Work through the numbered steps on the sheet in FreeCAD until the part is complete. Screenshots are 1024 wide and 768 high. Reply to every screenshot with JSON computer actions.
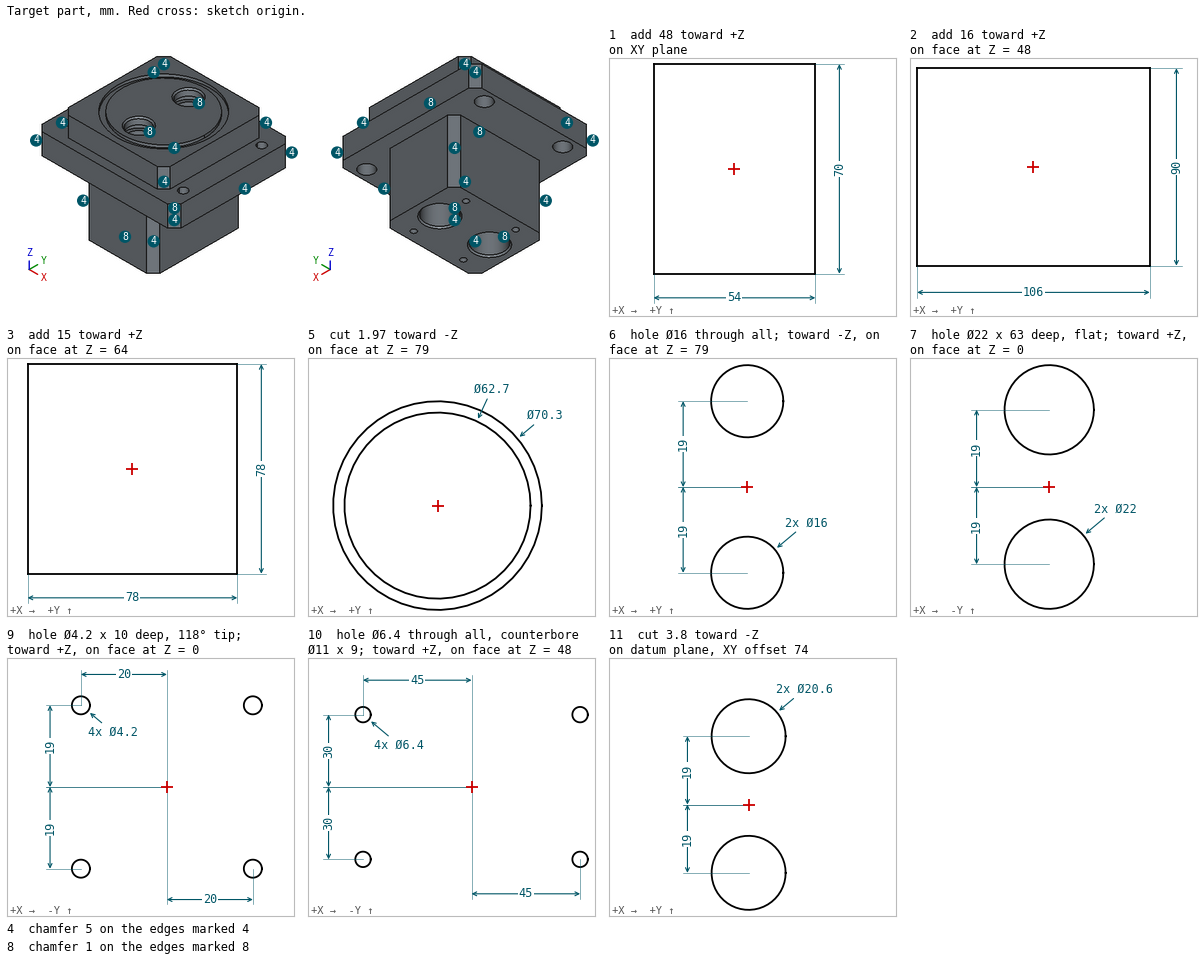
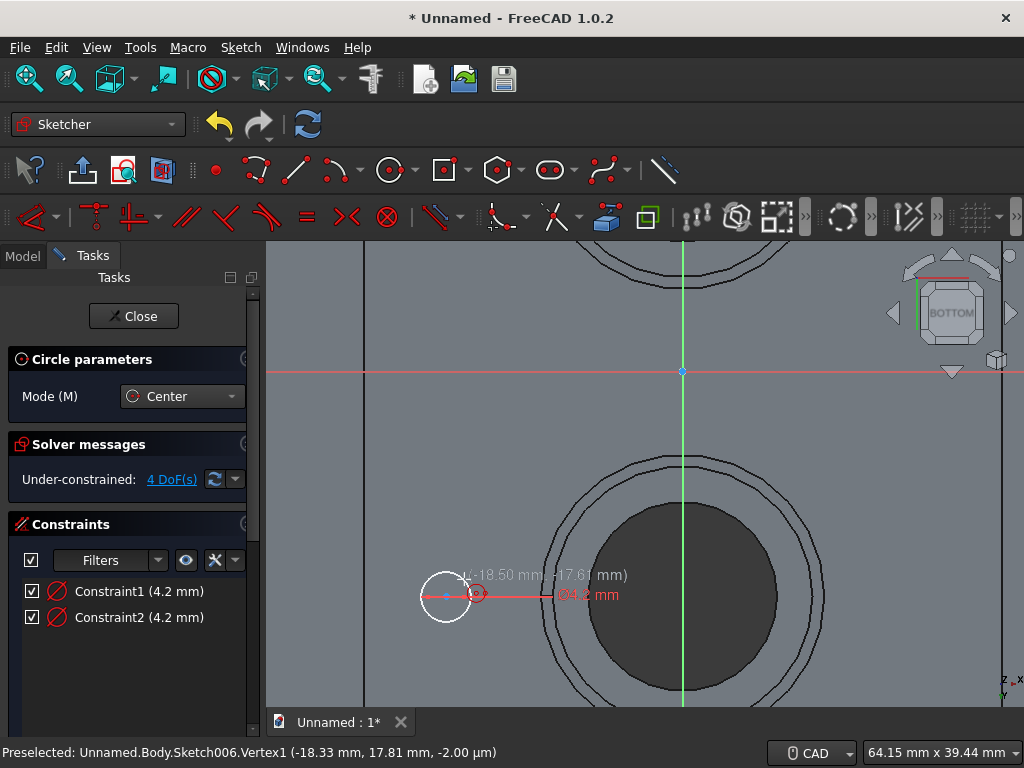
{"action": "scroll", "coordinate": [447, 598], "scroll_direction": "down", "scroll_amount": 3}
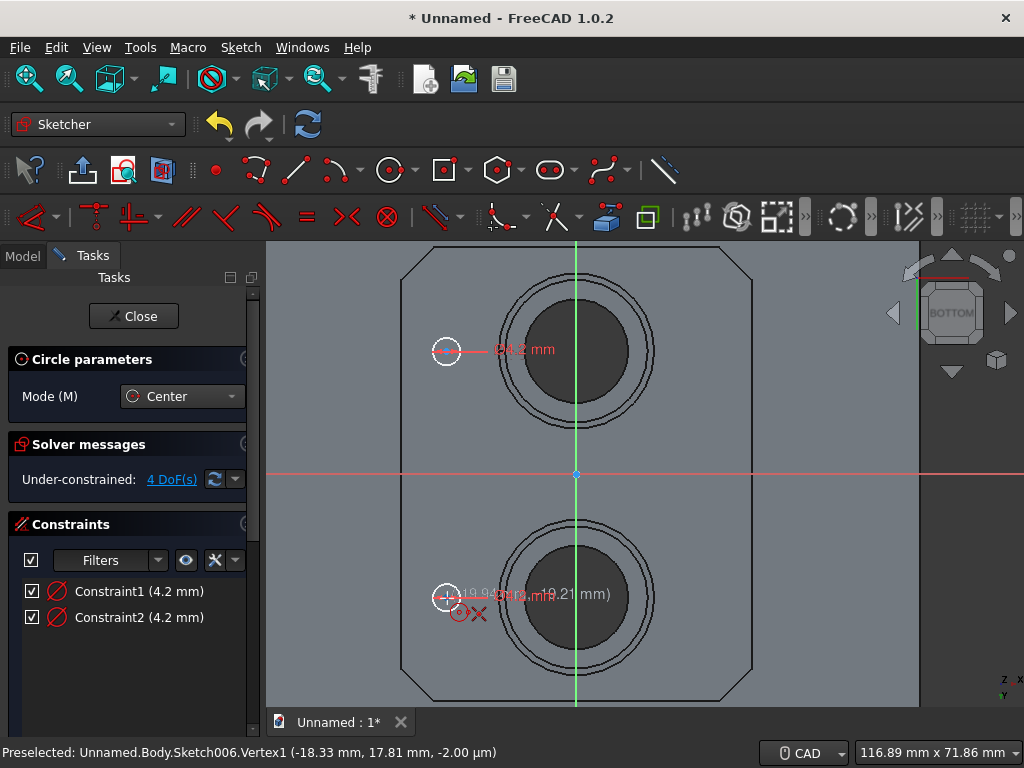
{"action": "scroll", "coordinate": [706, 598], "scroll_direction": "up", "scroll_amount": 3}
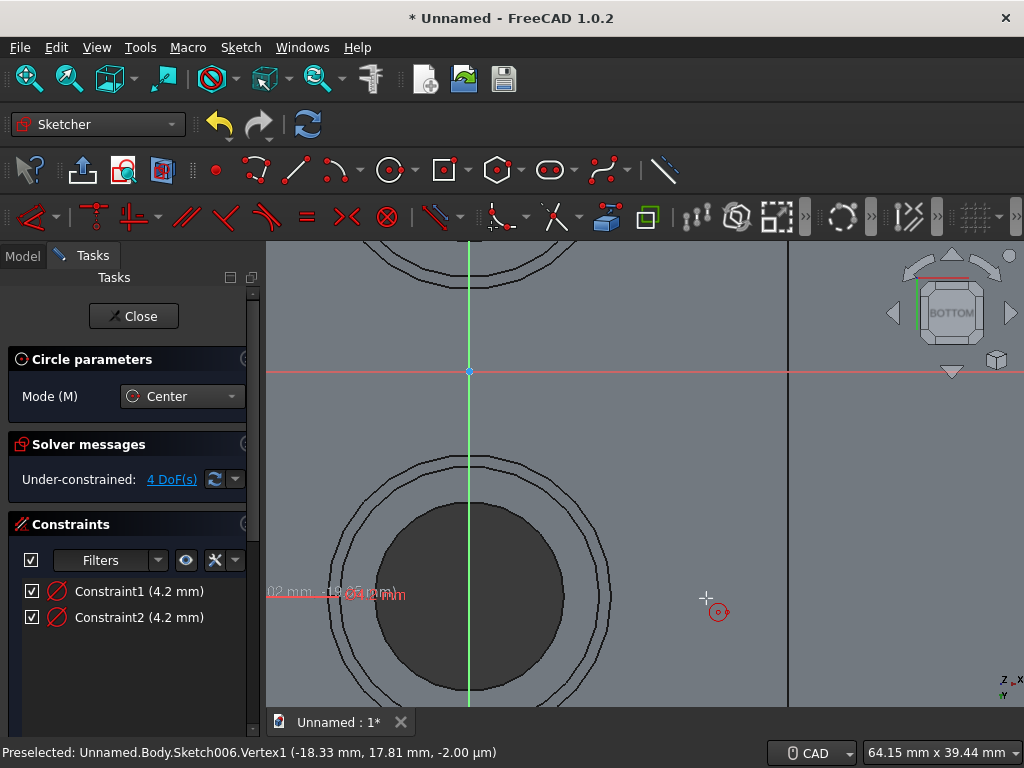
{"action": "left_click", "coordinate": [706, 596]}
{"action": "mouse_move", "coordinate": [723, 579]}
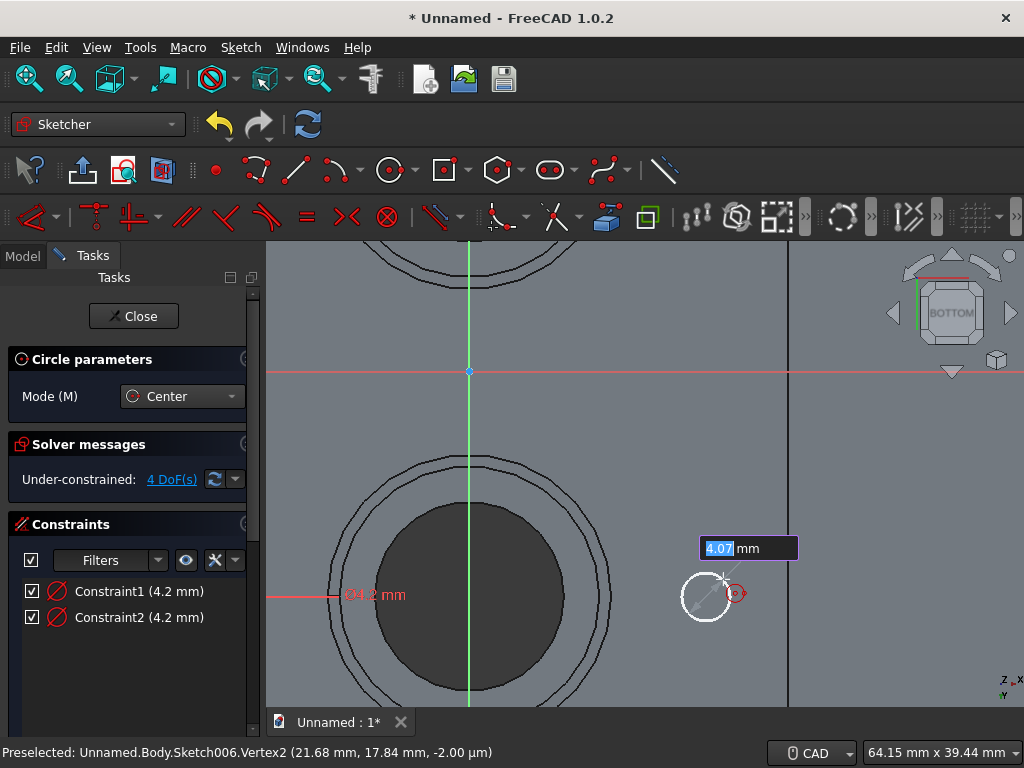
{"action": "type", "text": "4.2"}
{"action": "key", "text": "Return"}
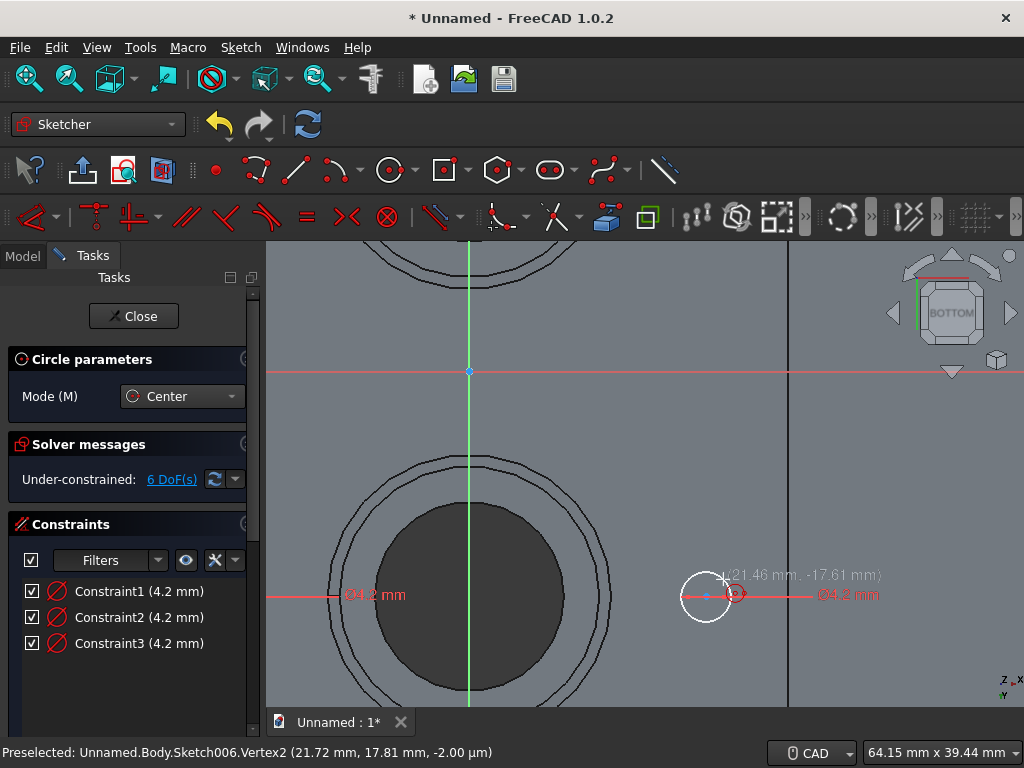
{"action": "scroll", "coordinate": [707, 598], "scroll_direction": "down", "scroll_amount": 3}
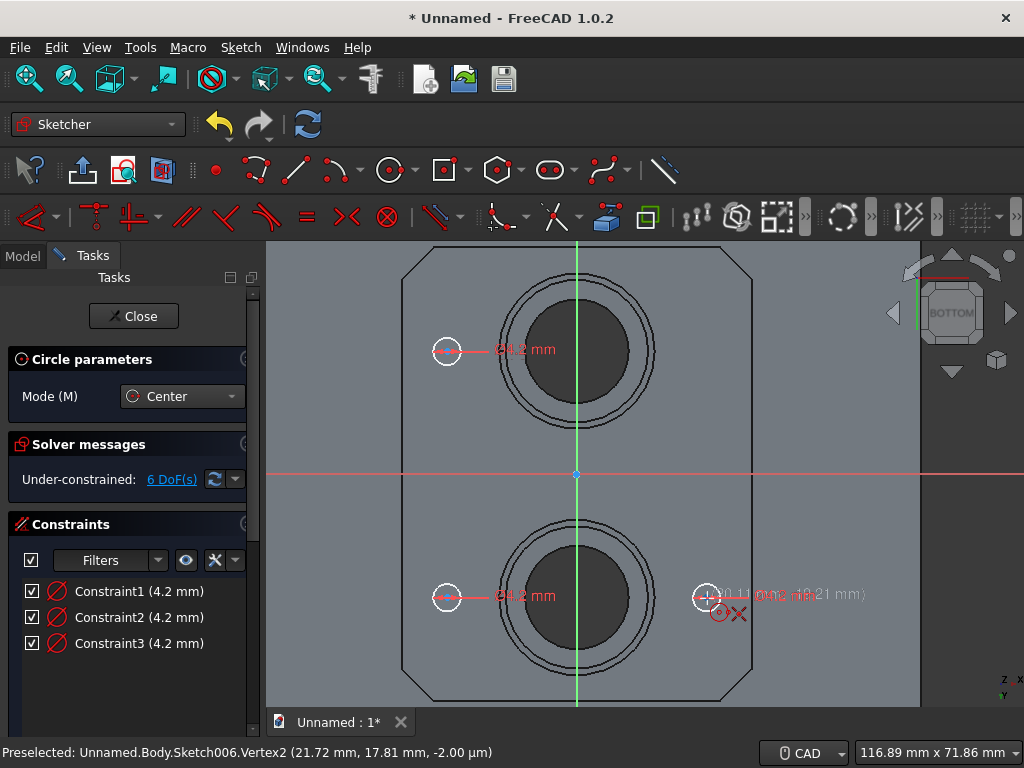
{"action": "scroll", "coordinate": [707, 351], "scroll_direction": "up", "scroll_amount": 3}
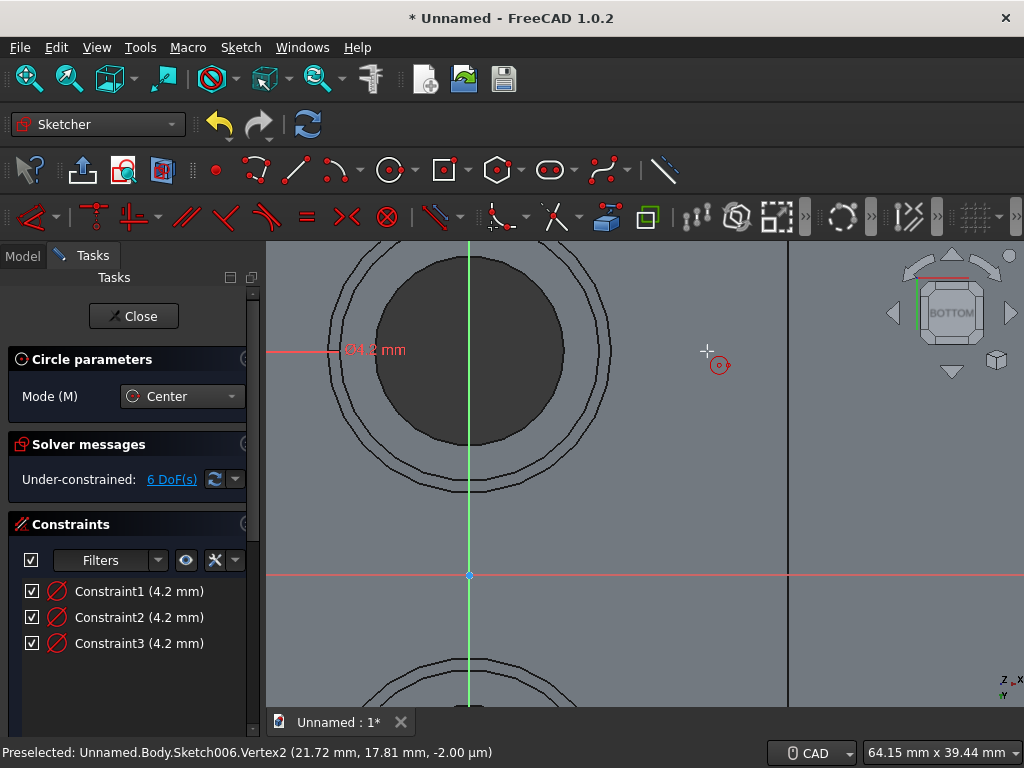
{"action": "left_click", "coordinate": [706, 351]}
{"action": "mouse_move", "coordinate": [723, 333]}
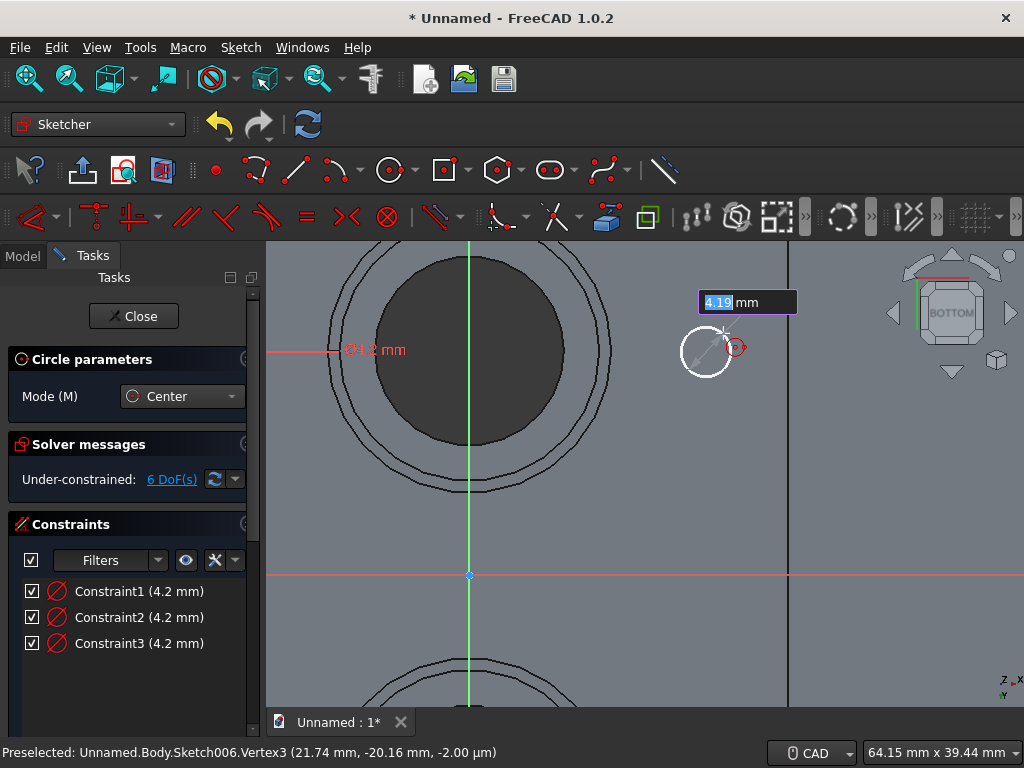
{"action": "type", "text": "4.2"}
{"action": "key", "text": "Return"}
{"action": "key", "text": "Escape"}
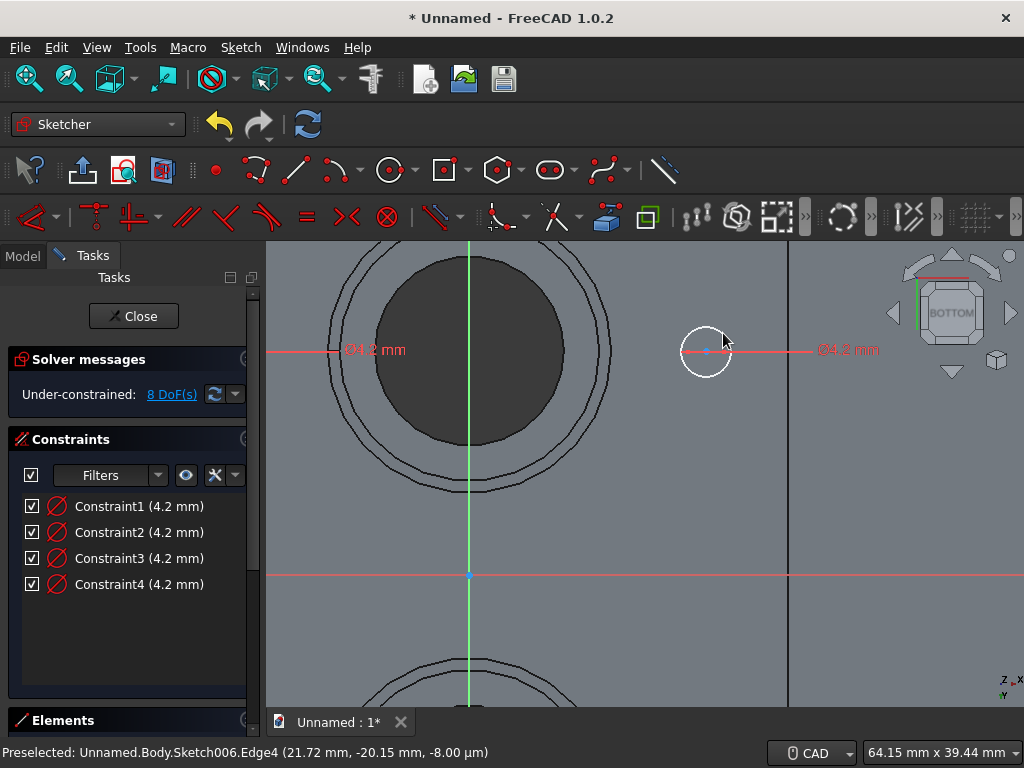
{"action": "scroll", "coordinate": [707, 351], "scroll_direction": "down", "scroll_amount": 3}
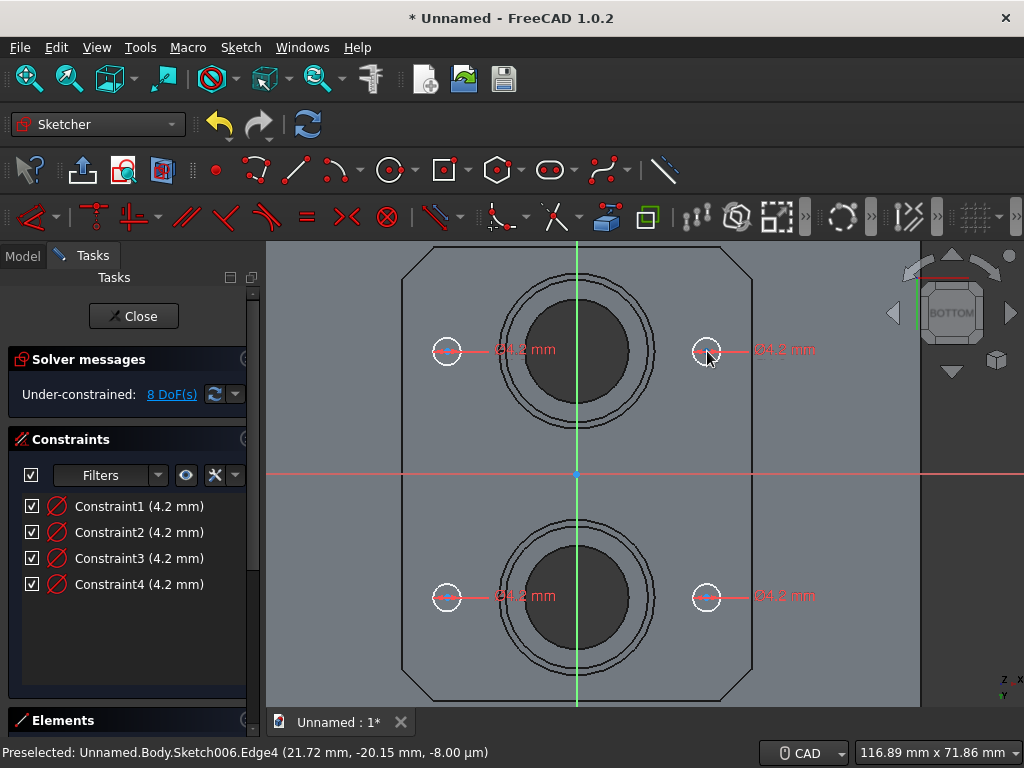
{"action": "left_click", "coordinate": [447, 352]}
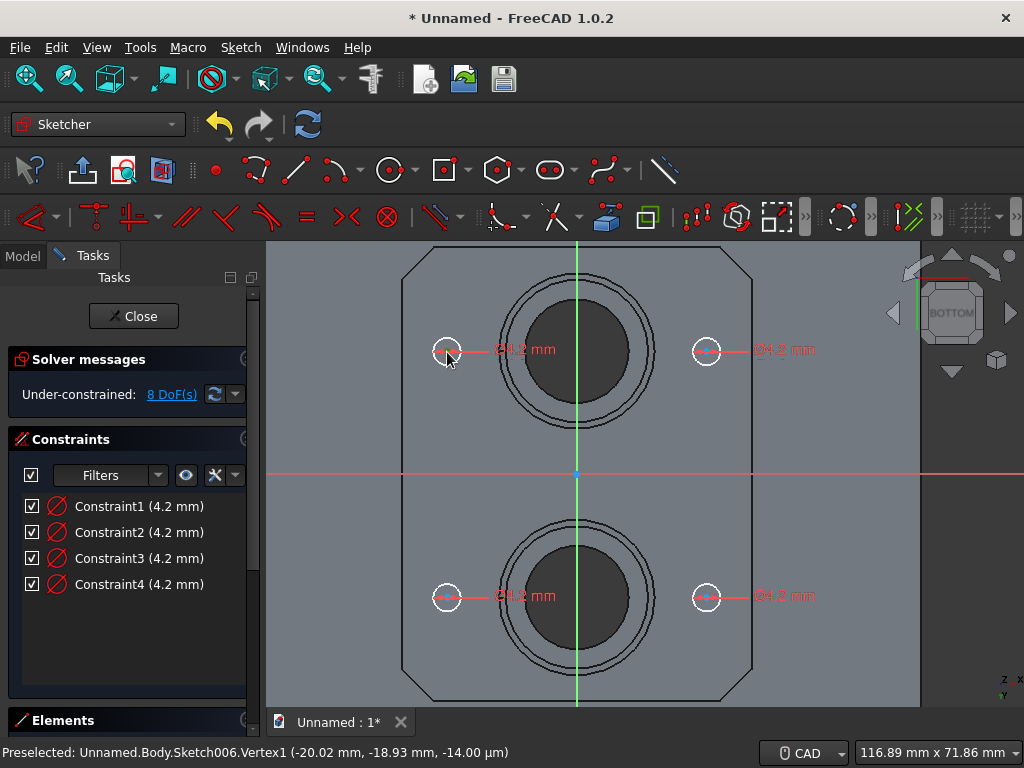
{"action": "left_click", "coordinate": [447, 598]}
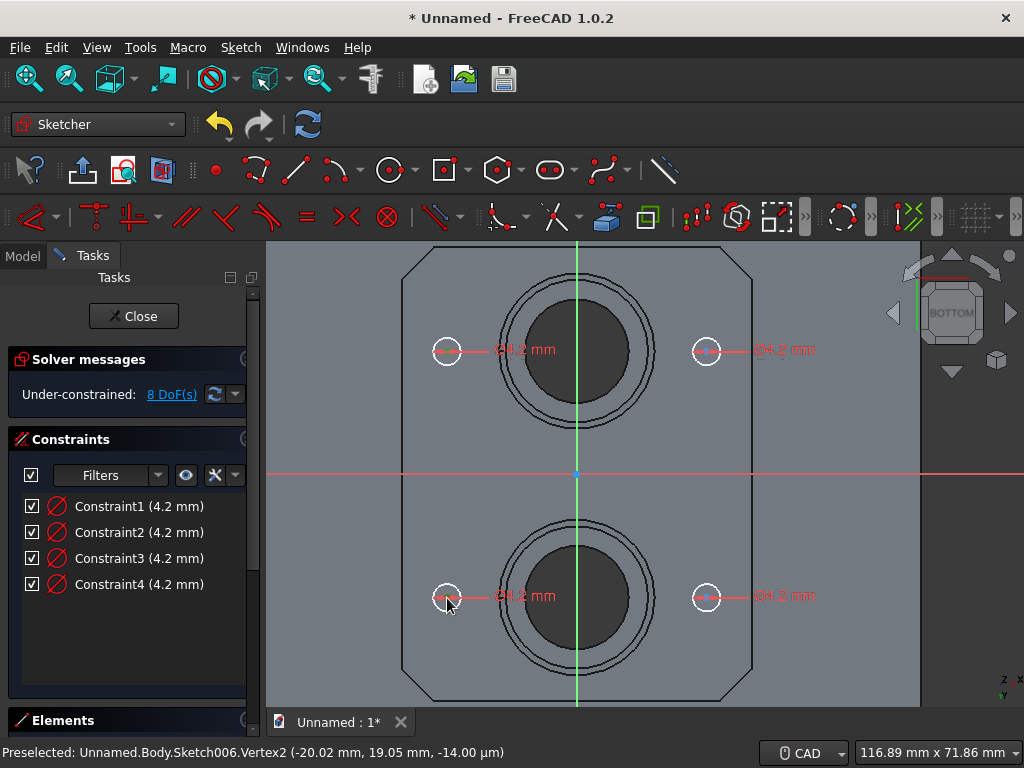
{"action": "key", "text": "v"}